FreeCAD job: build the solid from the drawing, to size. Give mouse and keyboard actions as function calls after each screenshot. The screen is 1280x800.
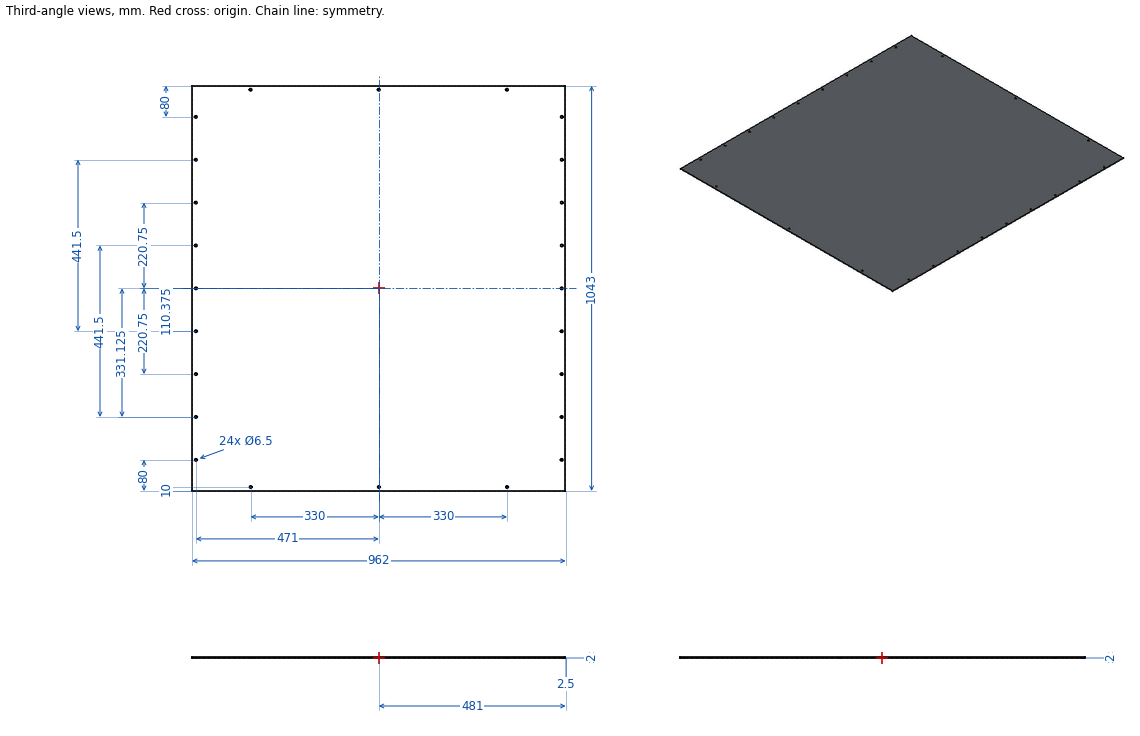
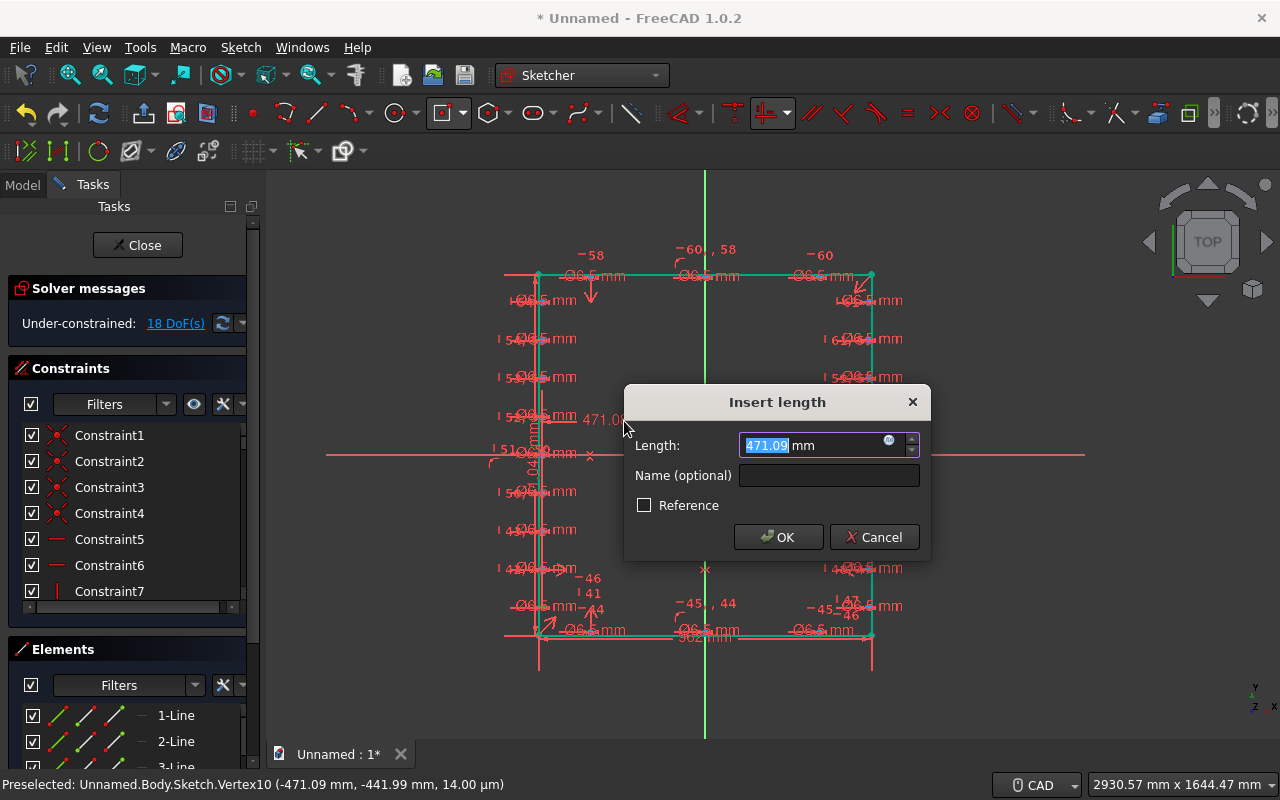
text(471)
key(Return)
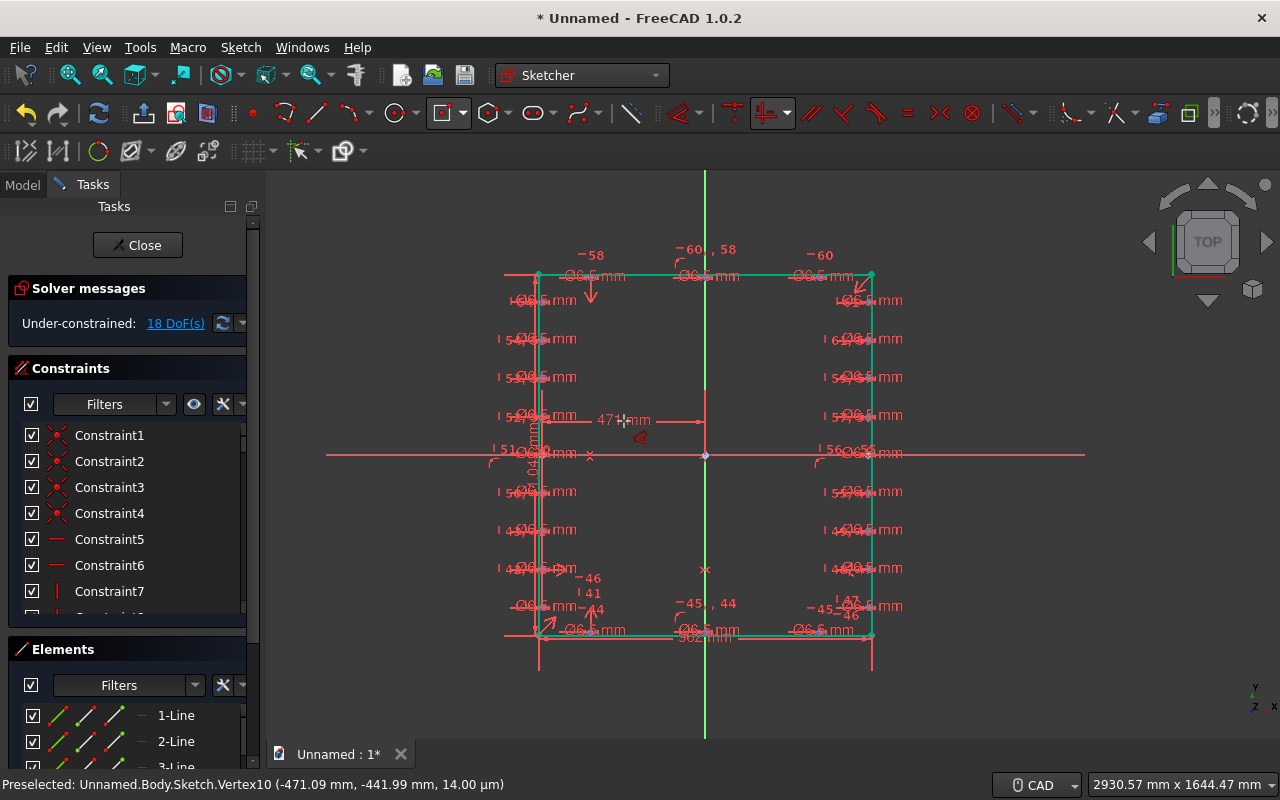
click(591, 632)
click(648, 666)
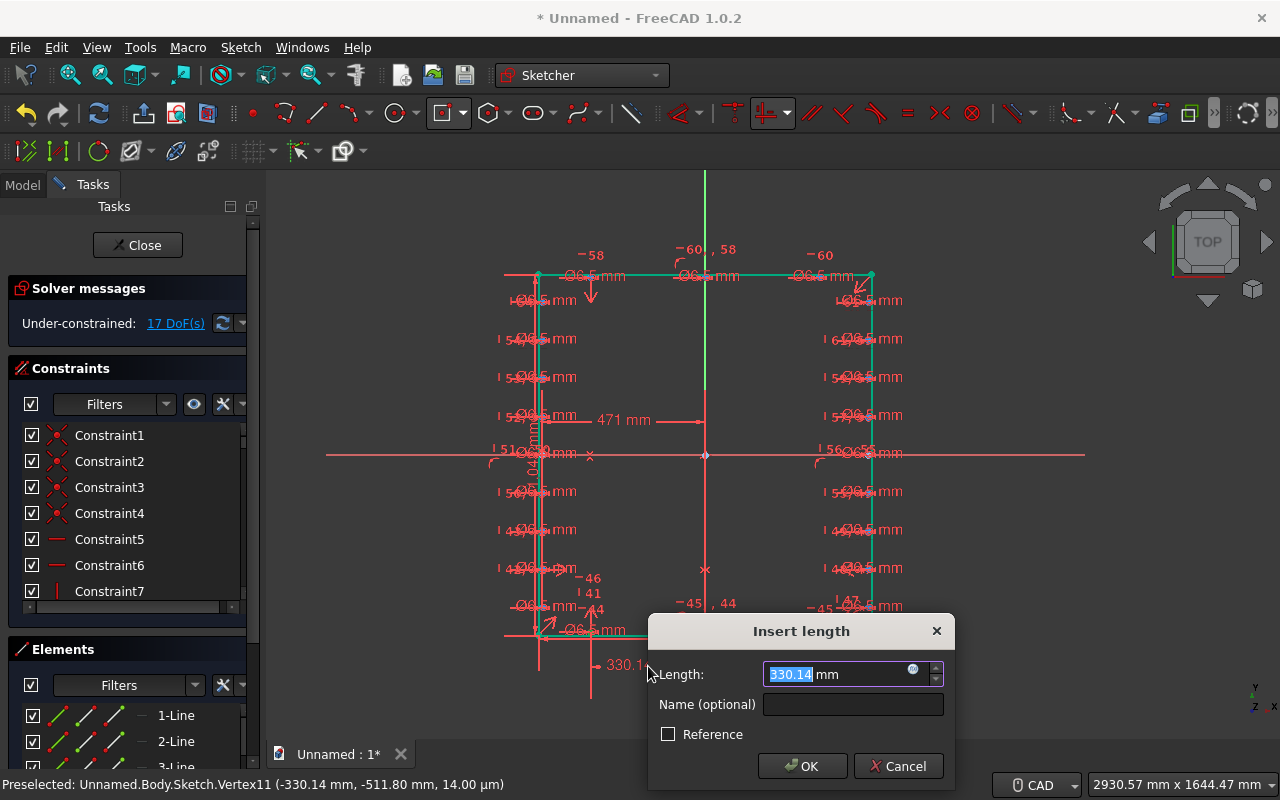
text(330)
key(Return)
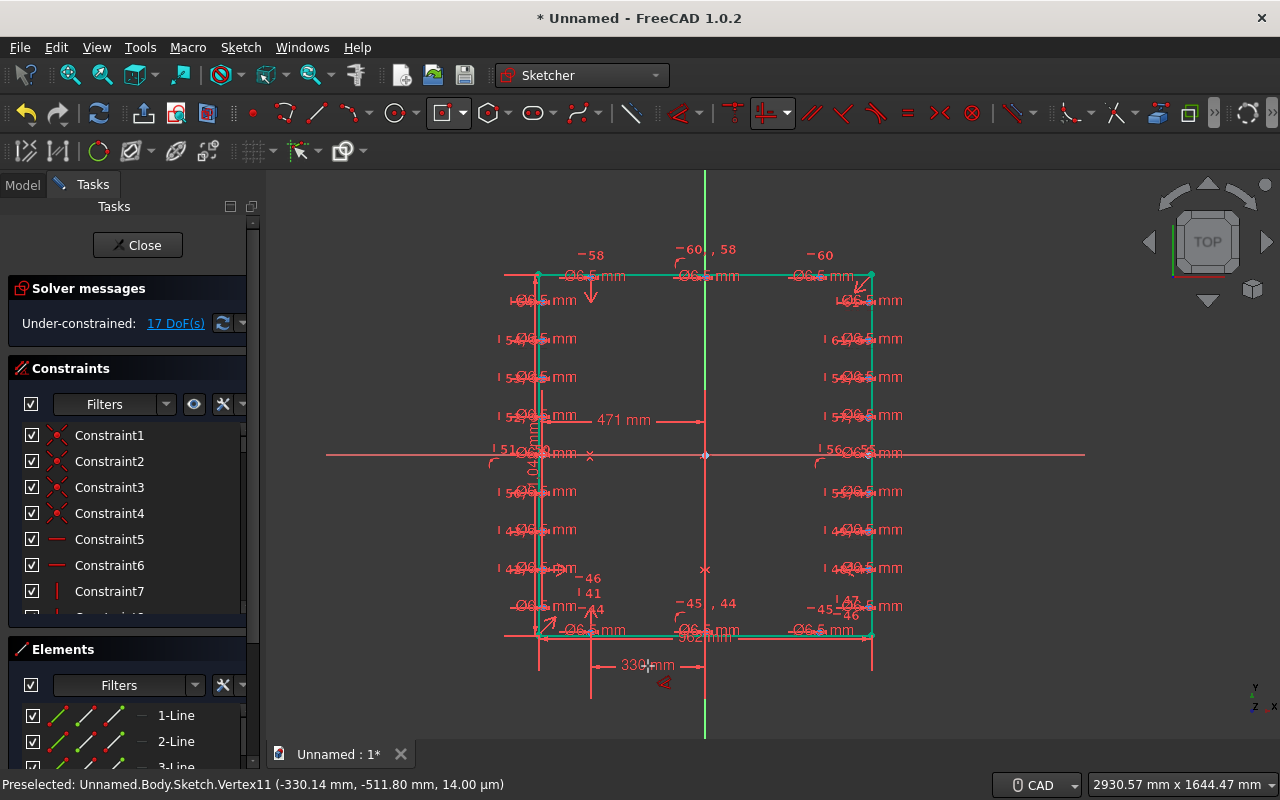
click(819, 632)
click(762, 666)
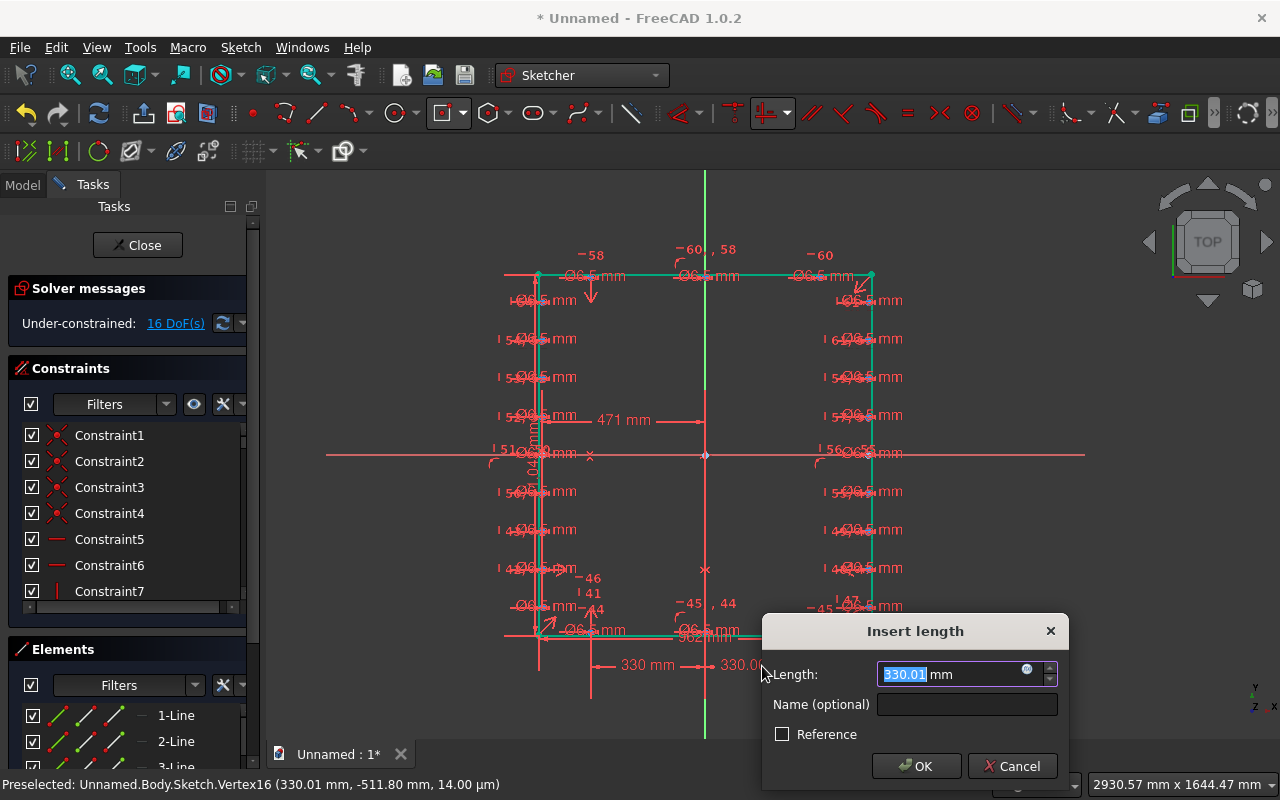
text(330)
key(Return)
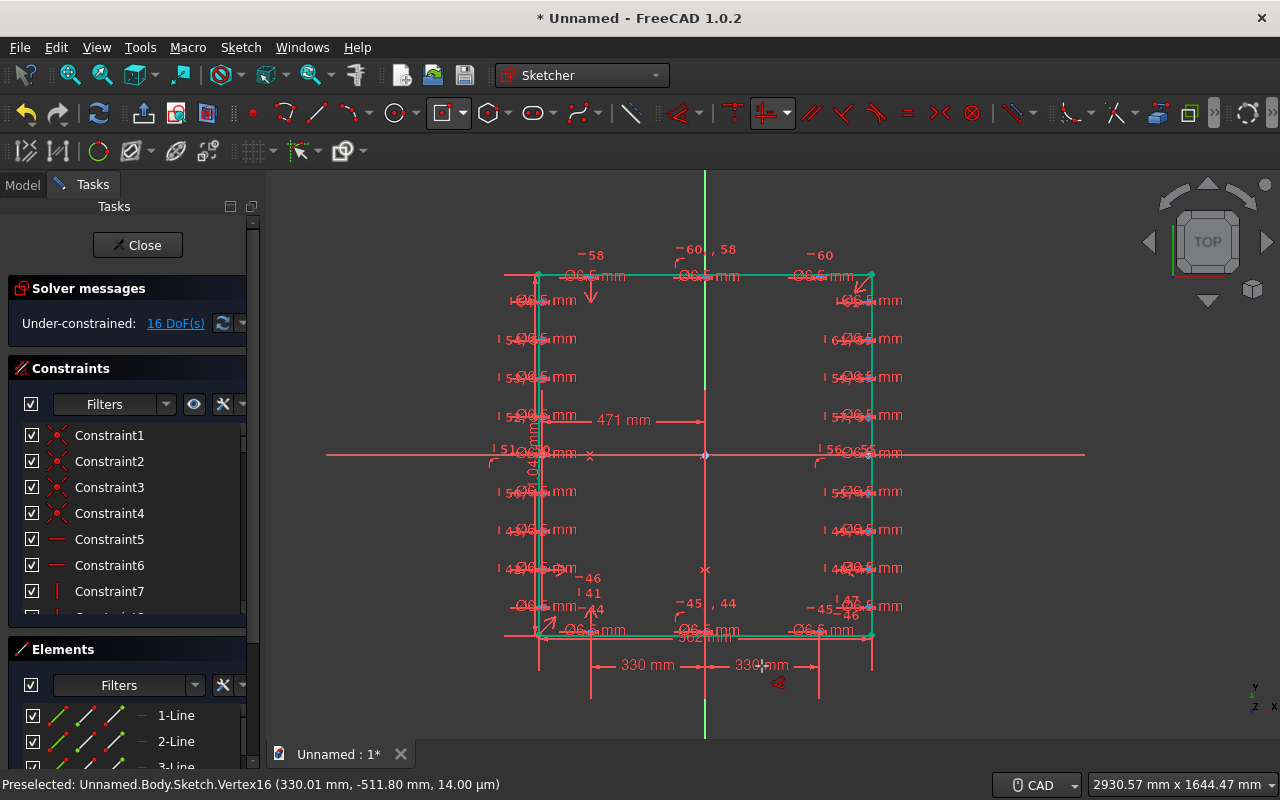
click(819, 278)
click(762, 244)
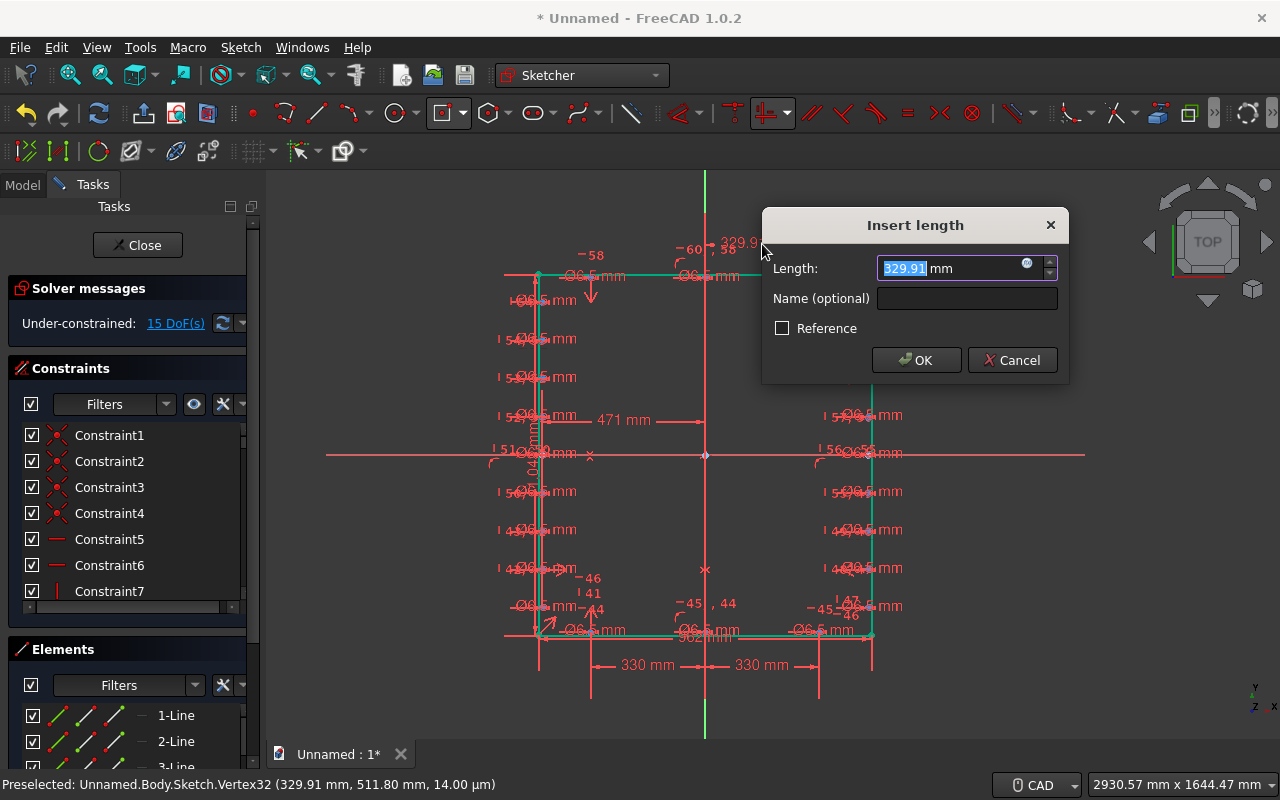
text(330)
key(Return)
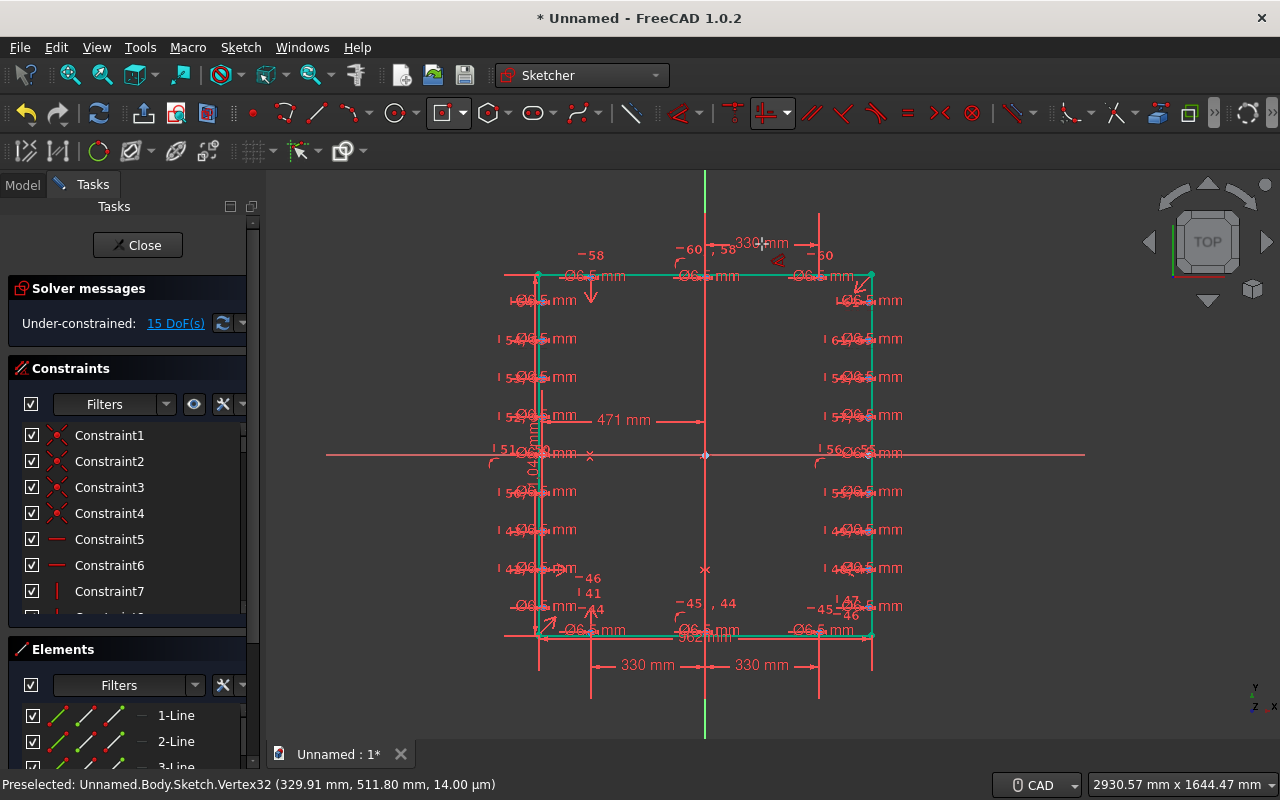
scroll(539, 636, up, 2)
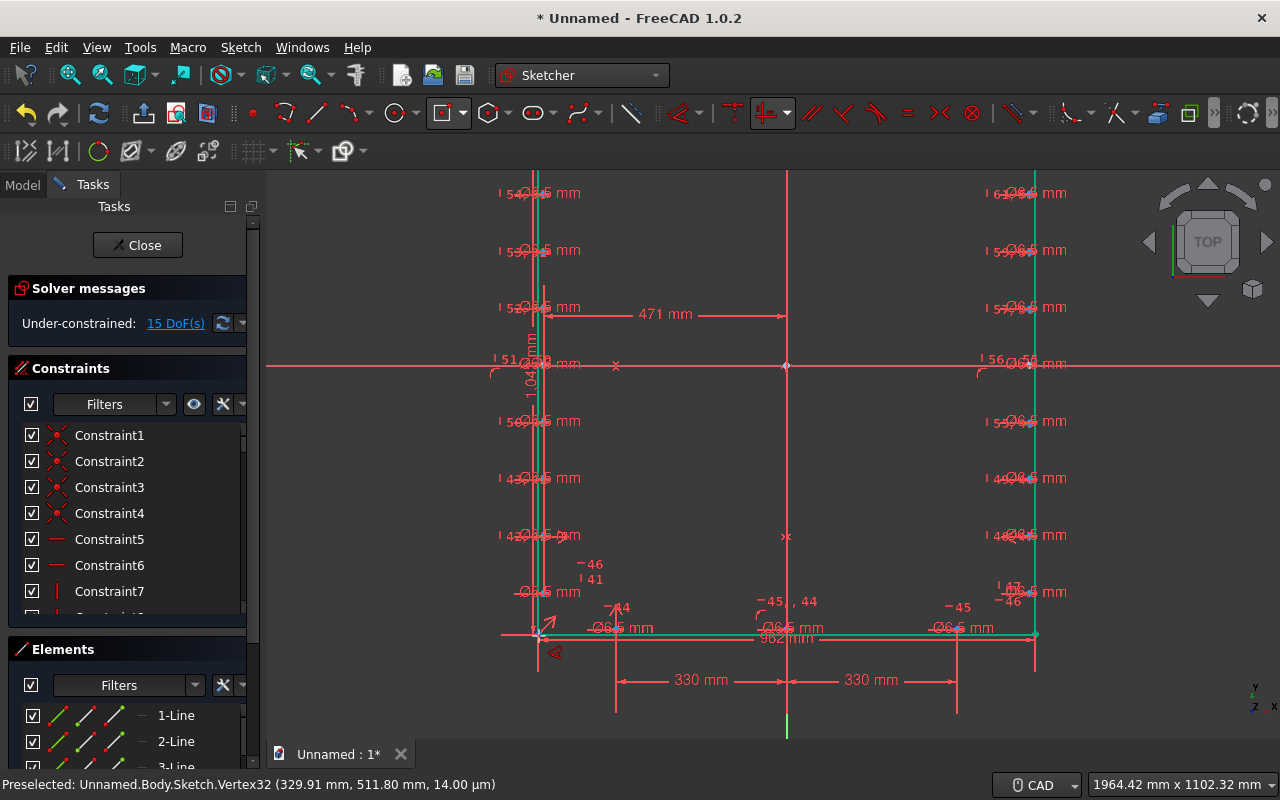
click(538, 635)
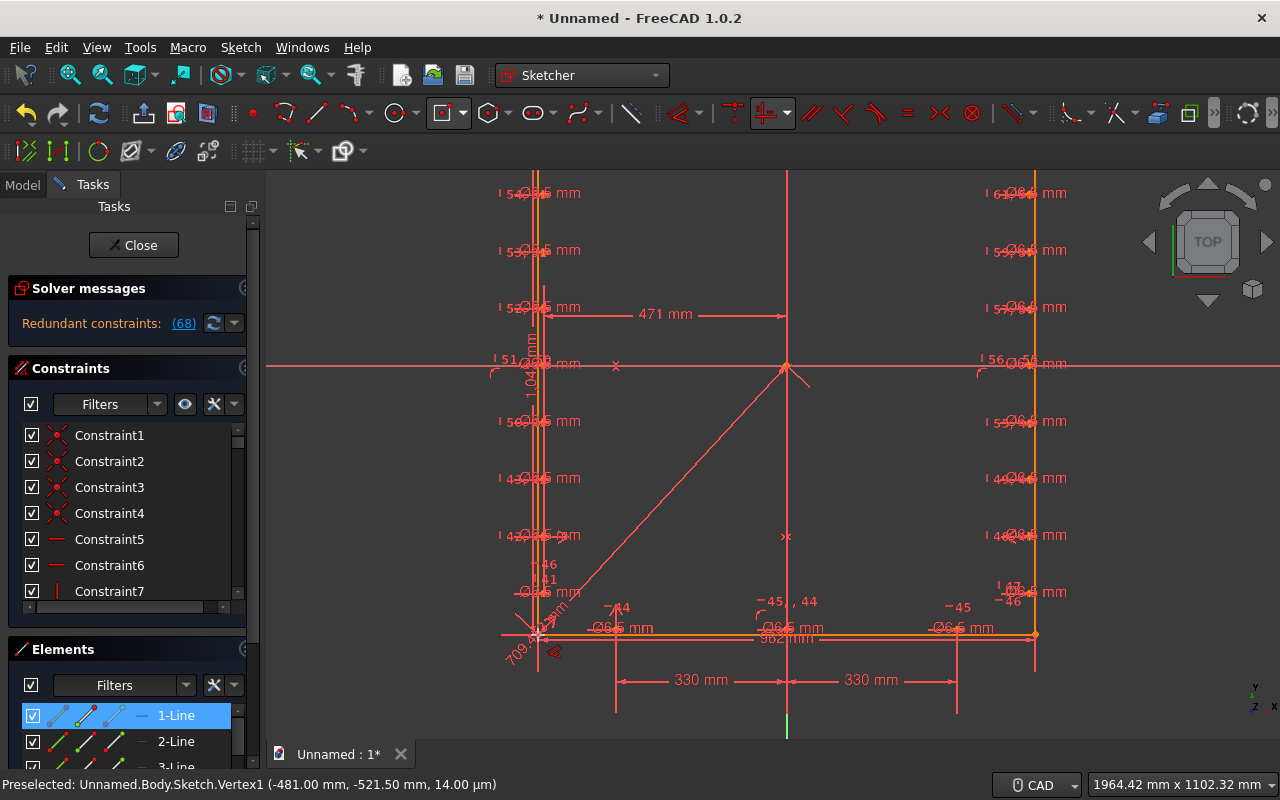
click(544, 594)
click(504, 614)